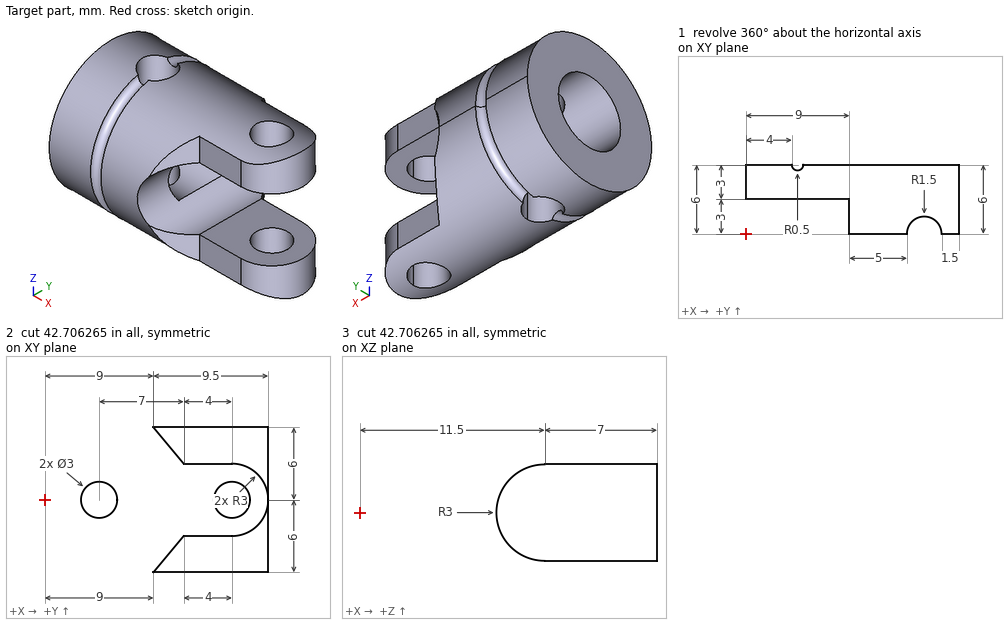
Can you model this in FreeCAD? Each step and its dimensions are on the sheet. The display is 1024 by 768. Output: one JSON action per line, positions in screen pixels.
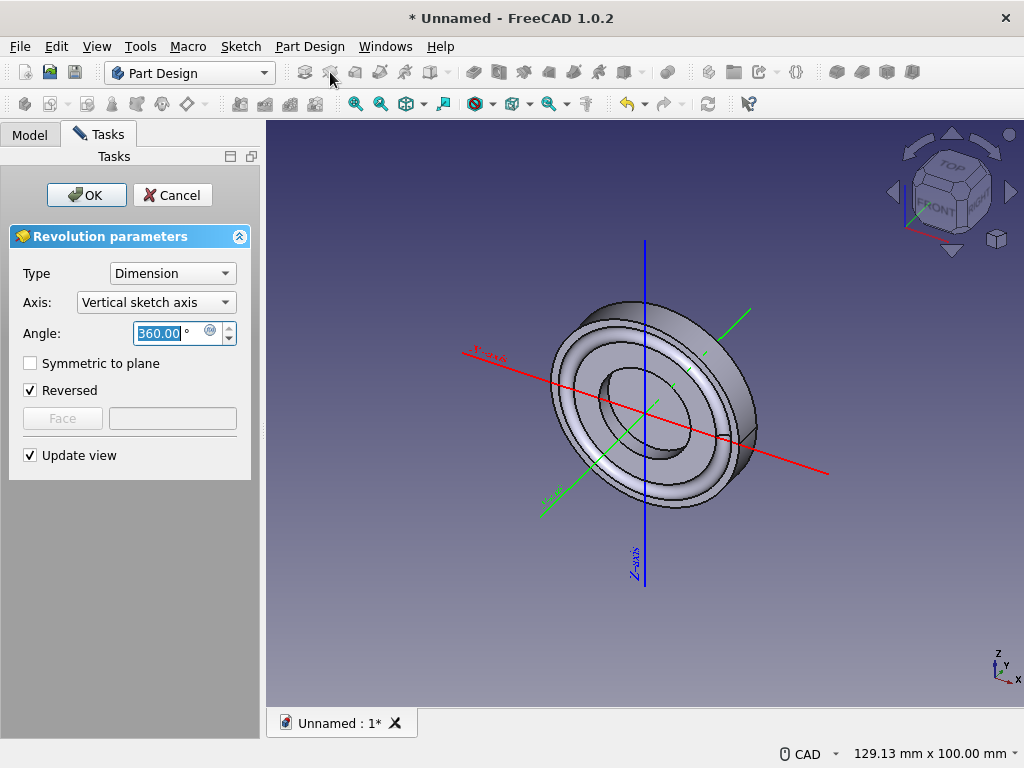
{"action": "left_click", "coordinate": [157, 302]}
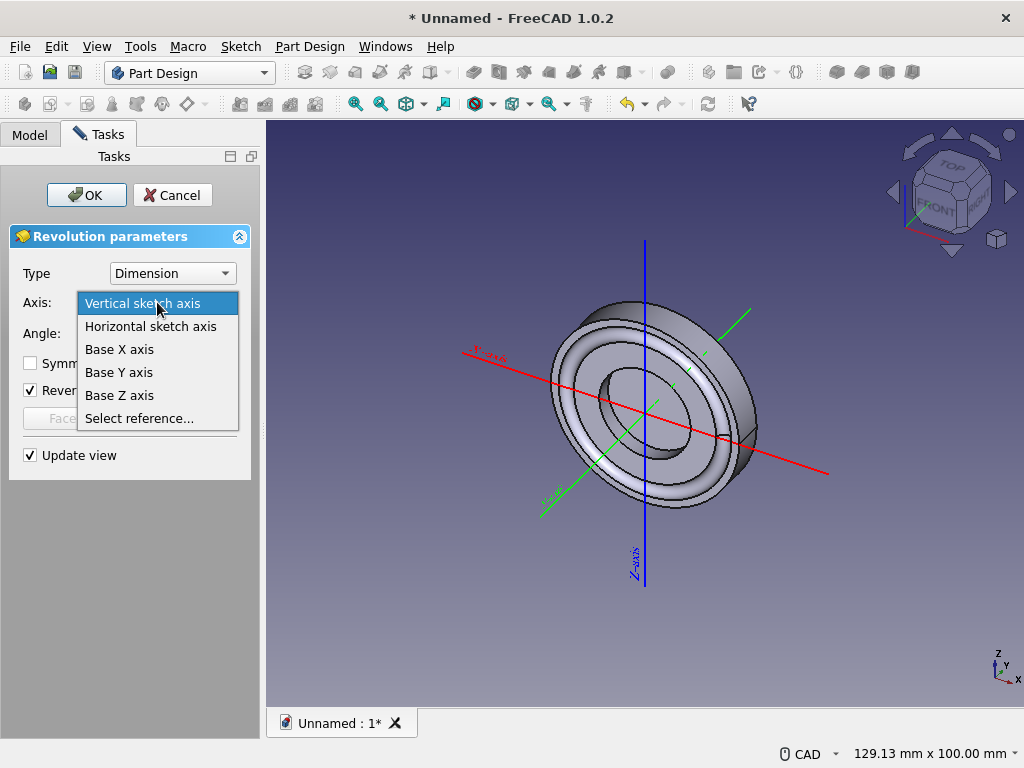
{"action": "left_click", "coordinate": [156, 326]}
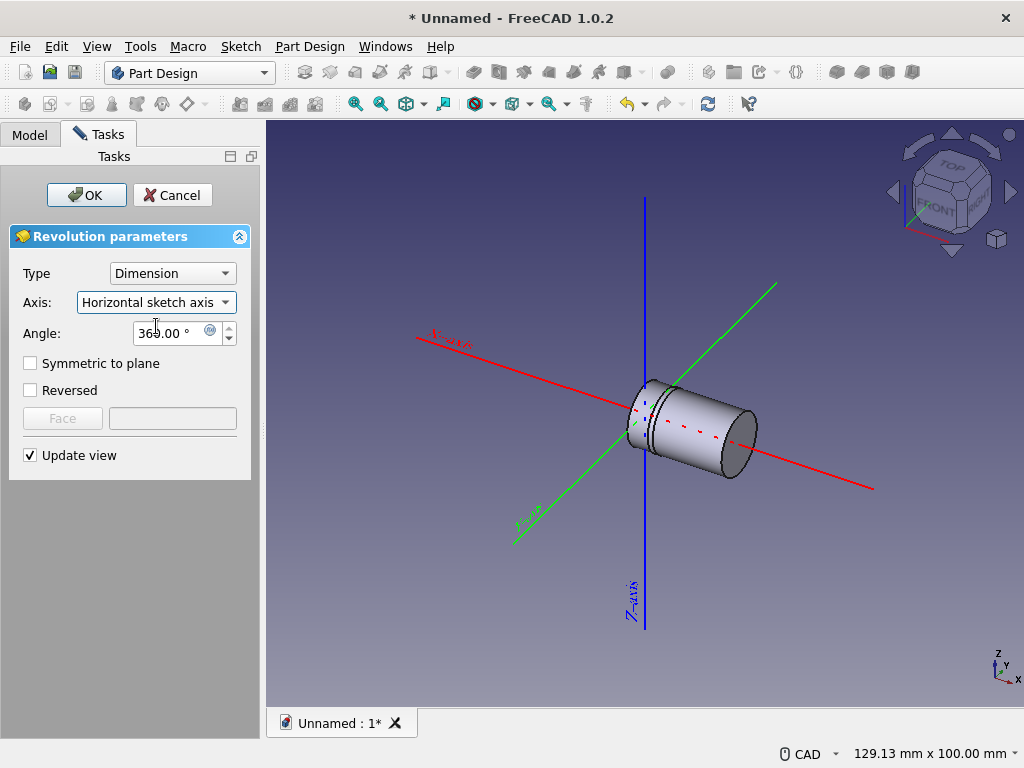
{"action": "left_click", "coordinate": [87, 195]}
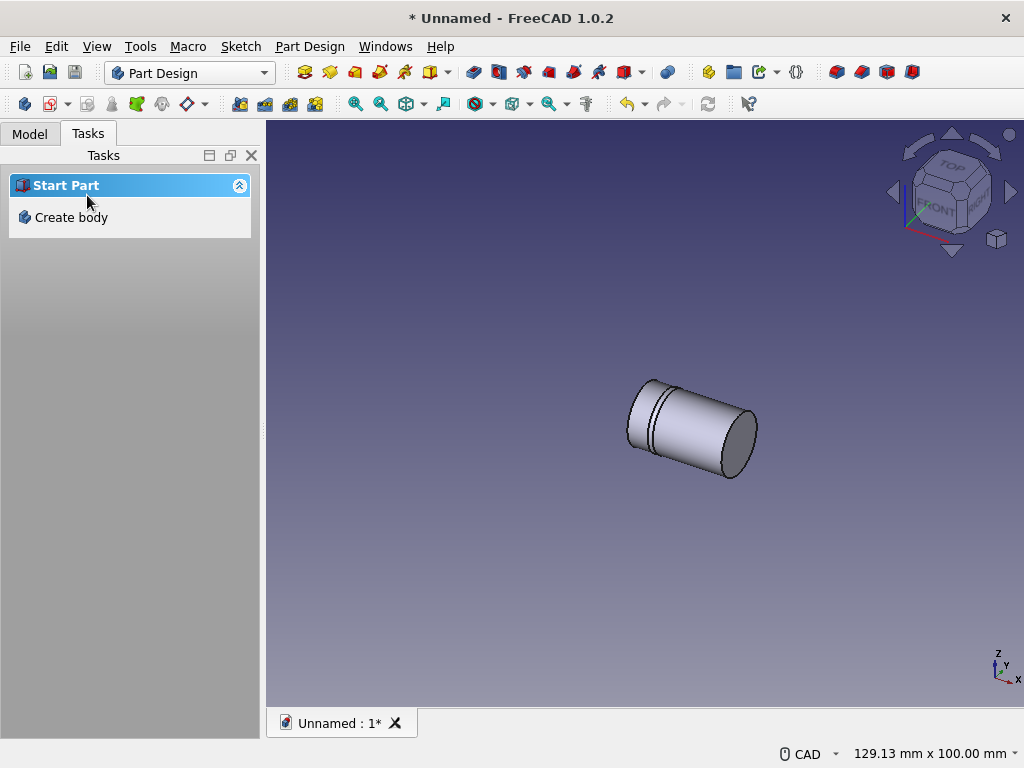
{"action": "left_click", "coordinate": [356, 104]}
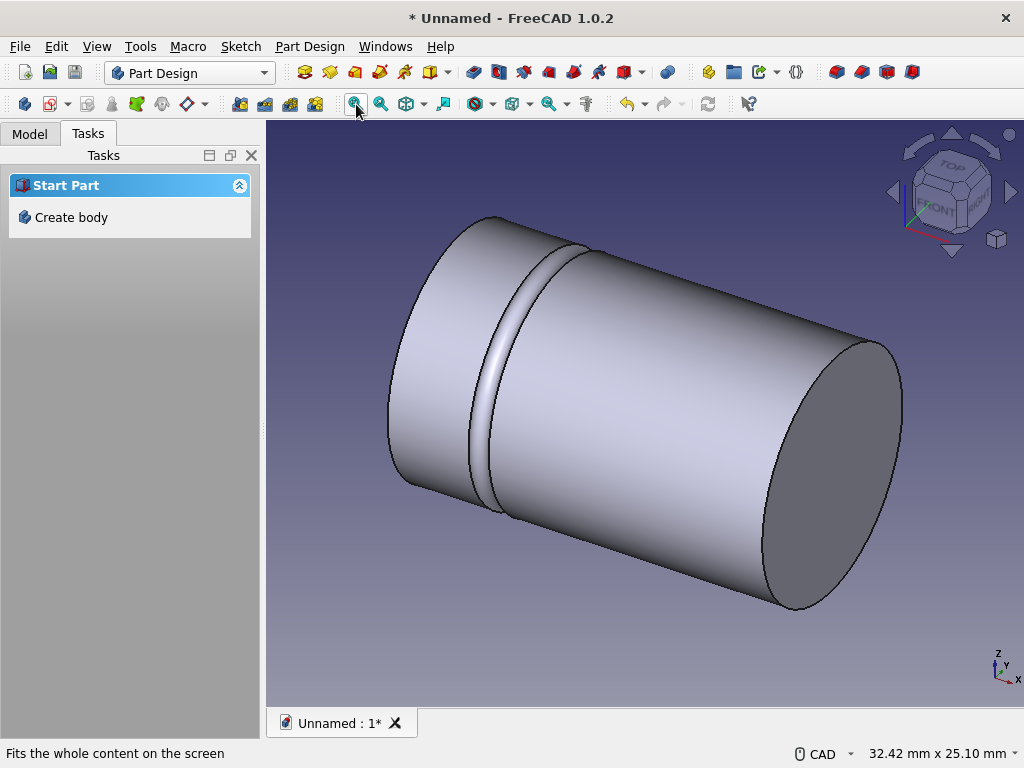
{"action": "left_click", "coordinate": [50, 104]}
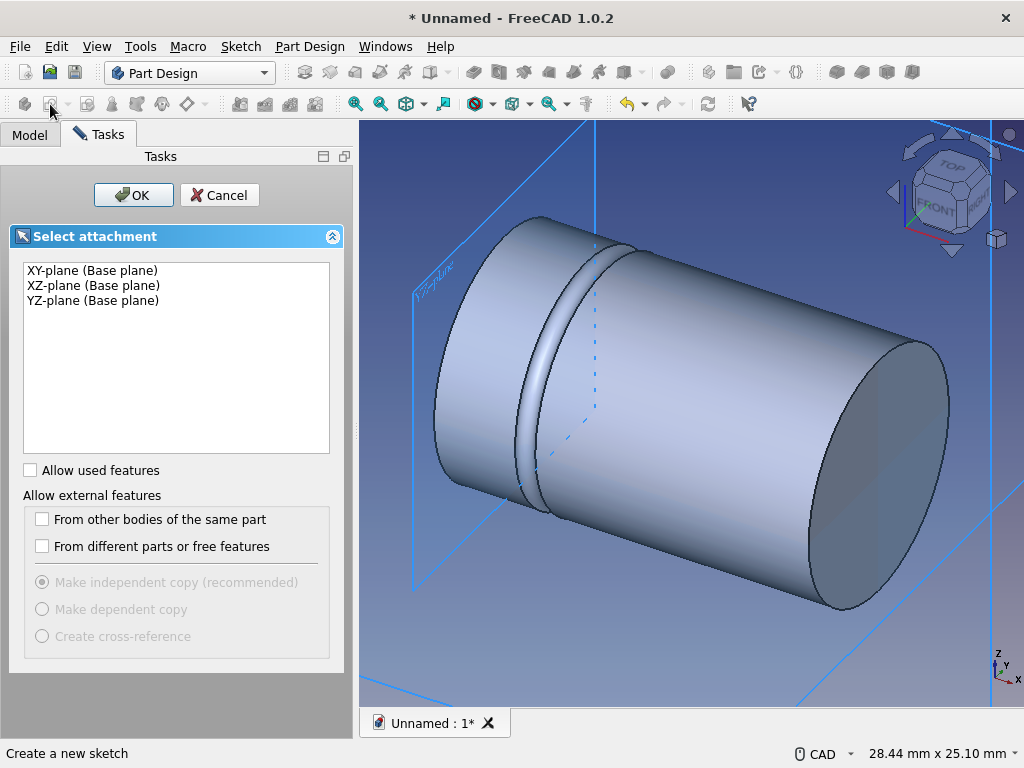
{"action": "left_click", "coordinate": [84, 270]}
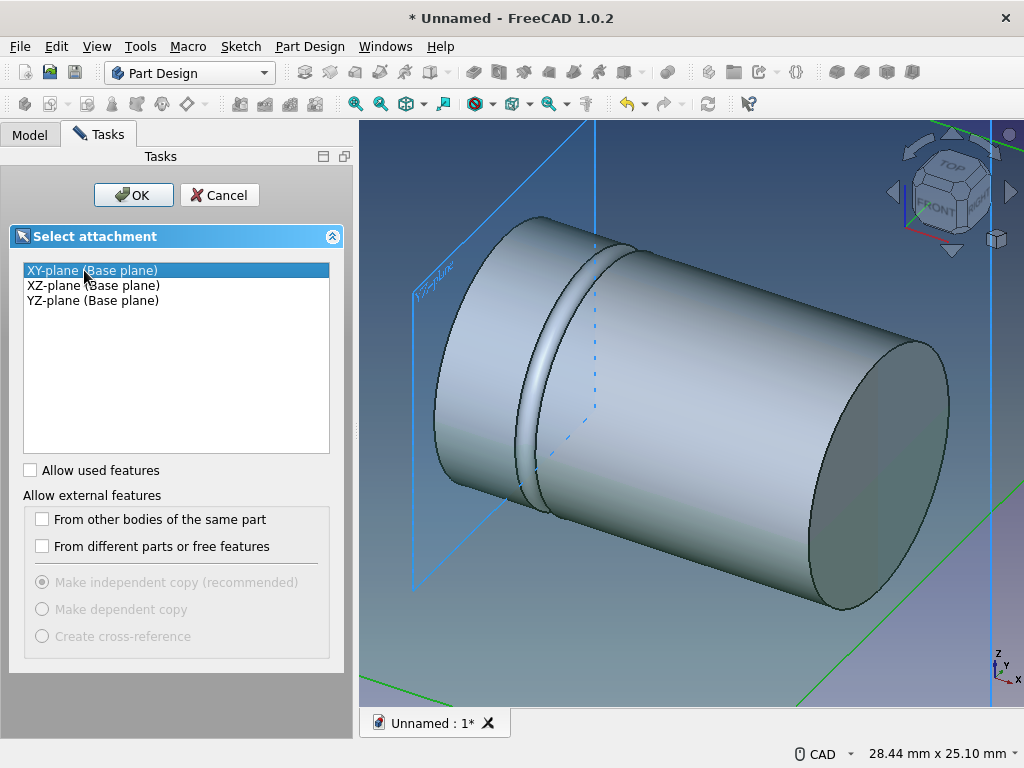
{"action": "left_click", "coordinate": [134, 195]}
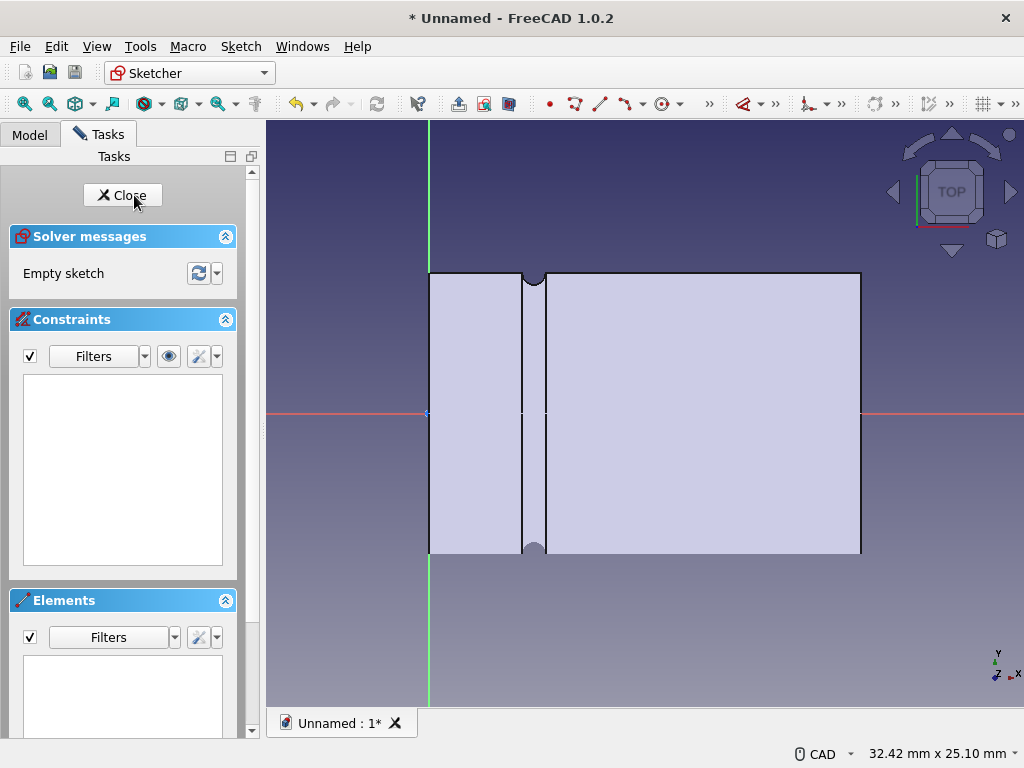
{"action": "left_click", "coordinate": [509, 104]}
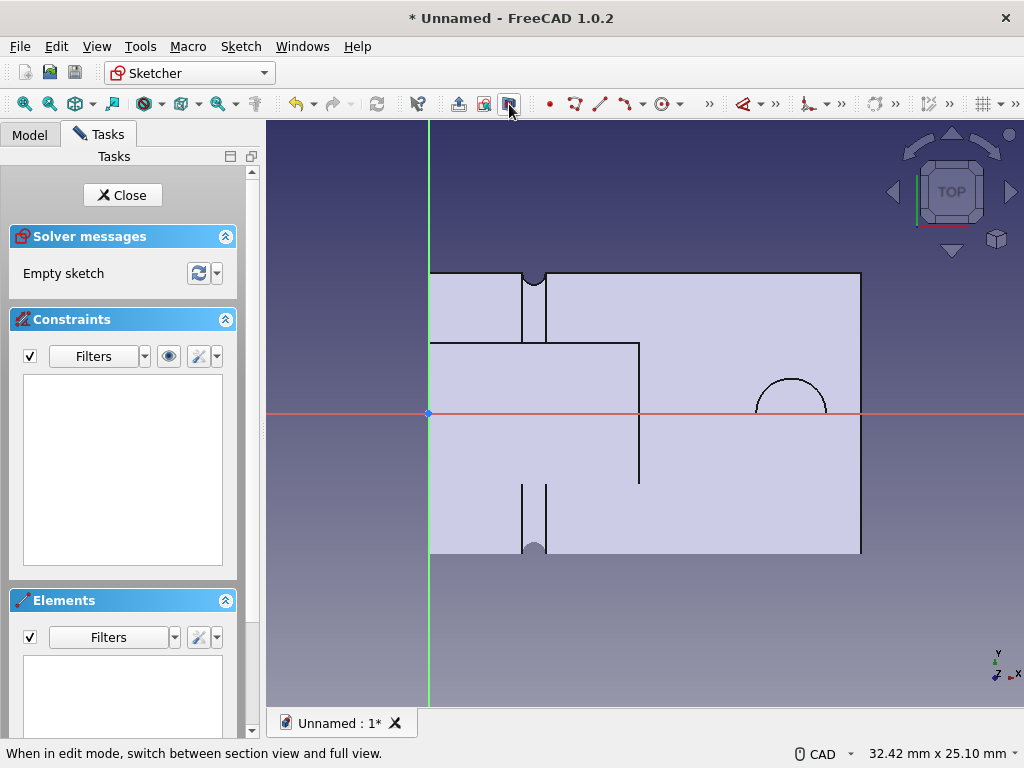
{"action": "scroll", "coordinate": [294, 413], "scroll_direction": "down", "scroll_amount": 1}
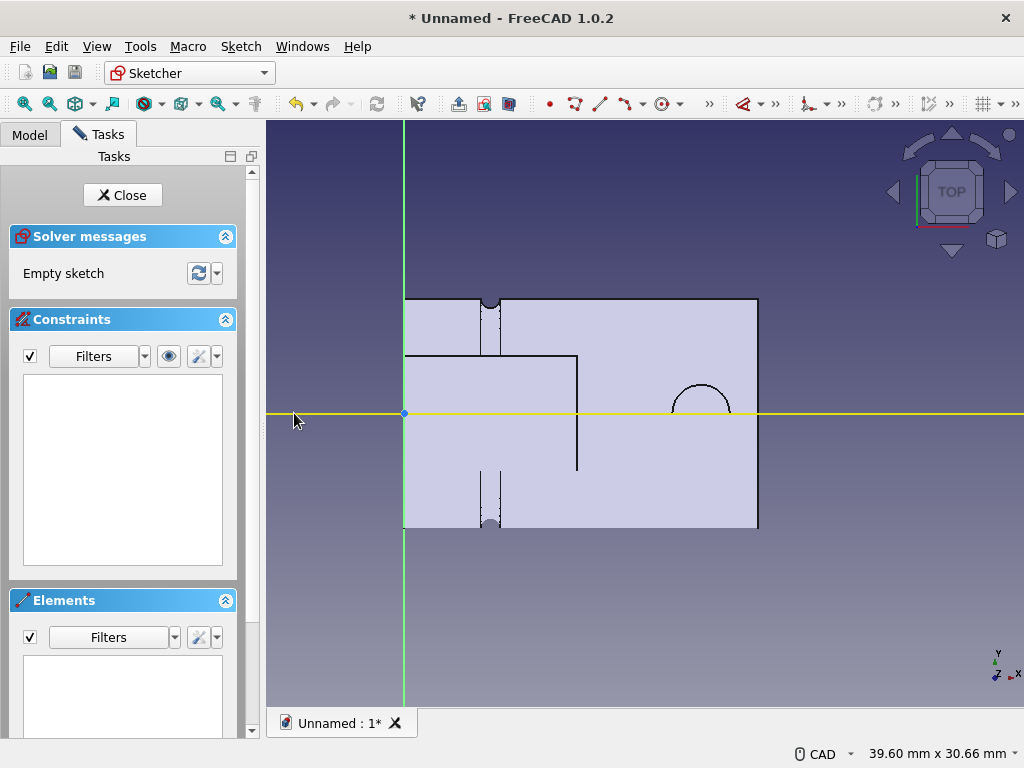
{"action": "left_click", "coordinate": [575, 104]}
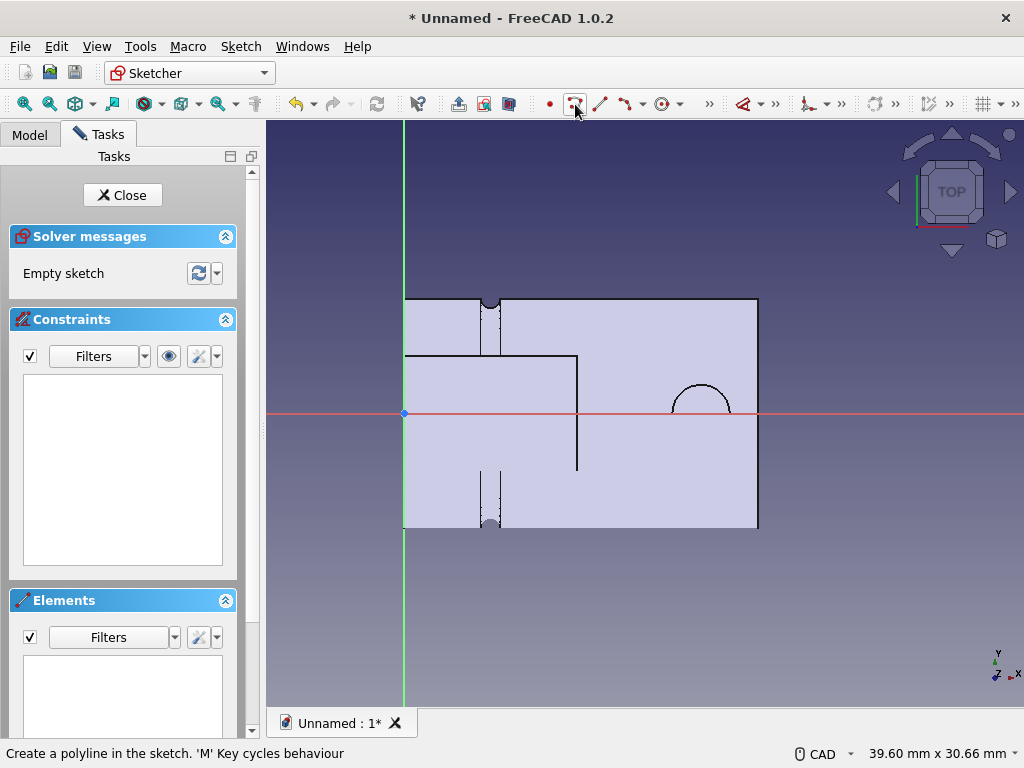
{"action": "left_click", "coordinate": [758, 414]}
{"action": "left_click", "coordinate": [758, 299]}
{"action": "left_click", "coordinate": [577, 299]}
{"action": "left_click", "coordinate": [624, 356]}
{"action": "left_click", "coordinate": [701, 356]}
{"action": "right_click", "coordinate": [701, 356]}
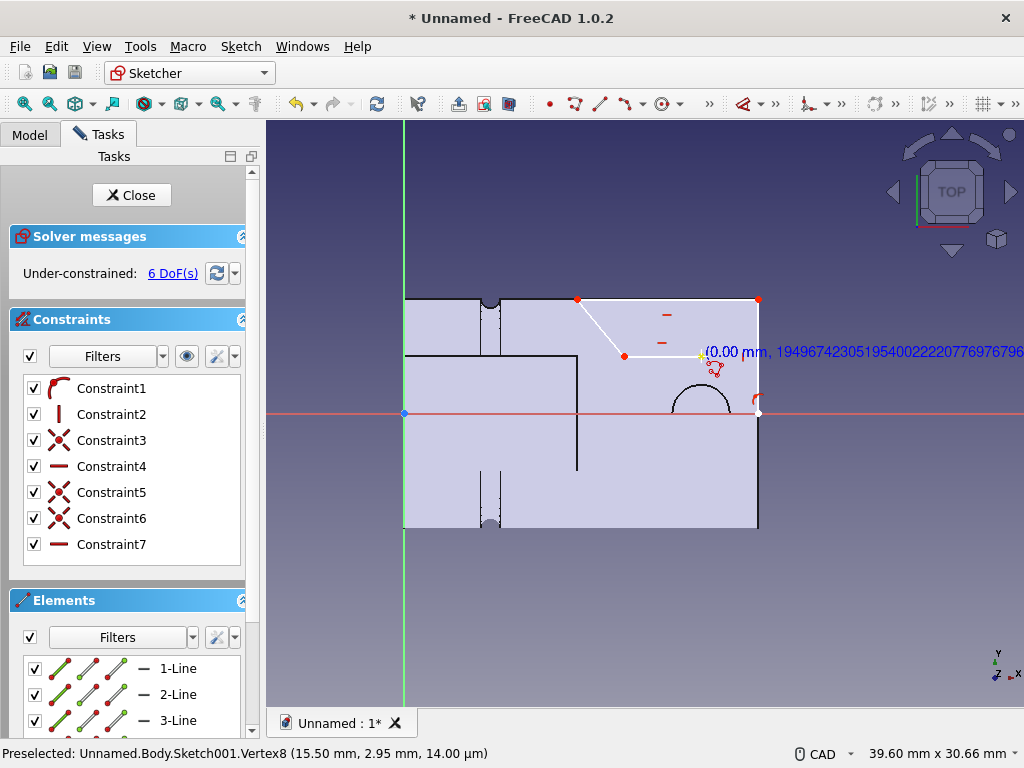
{"action": "left_click", "coordinate": [624, 104]}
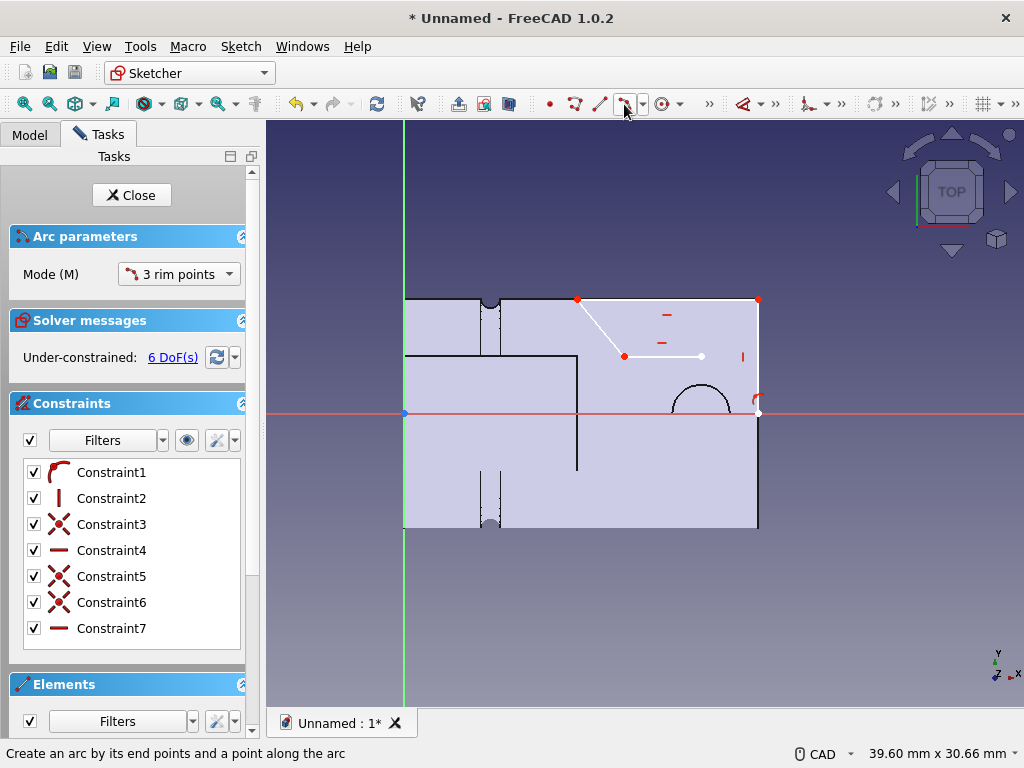
{"action": "left_click", "coordinate": [701, 357]}
{"action": "left_click", "coordinate": [758, 414]}
{"action": "left_click", "coordinate": [742, 373]}